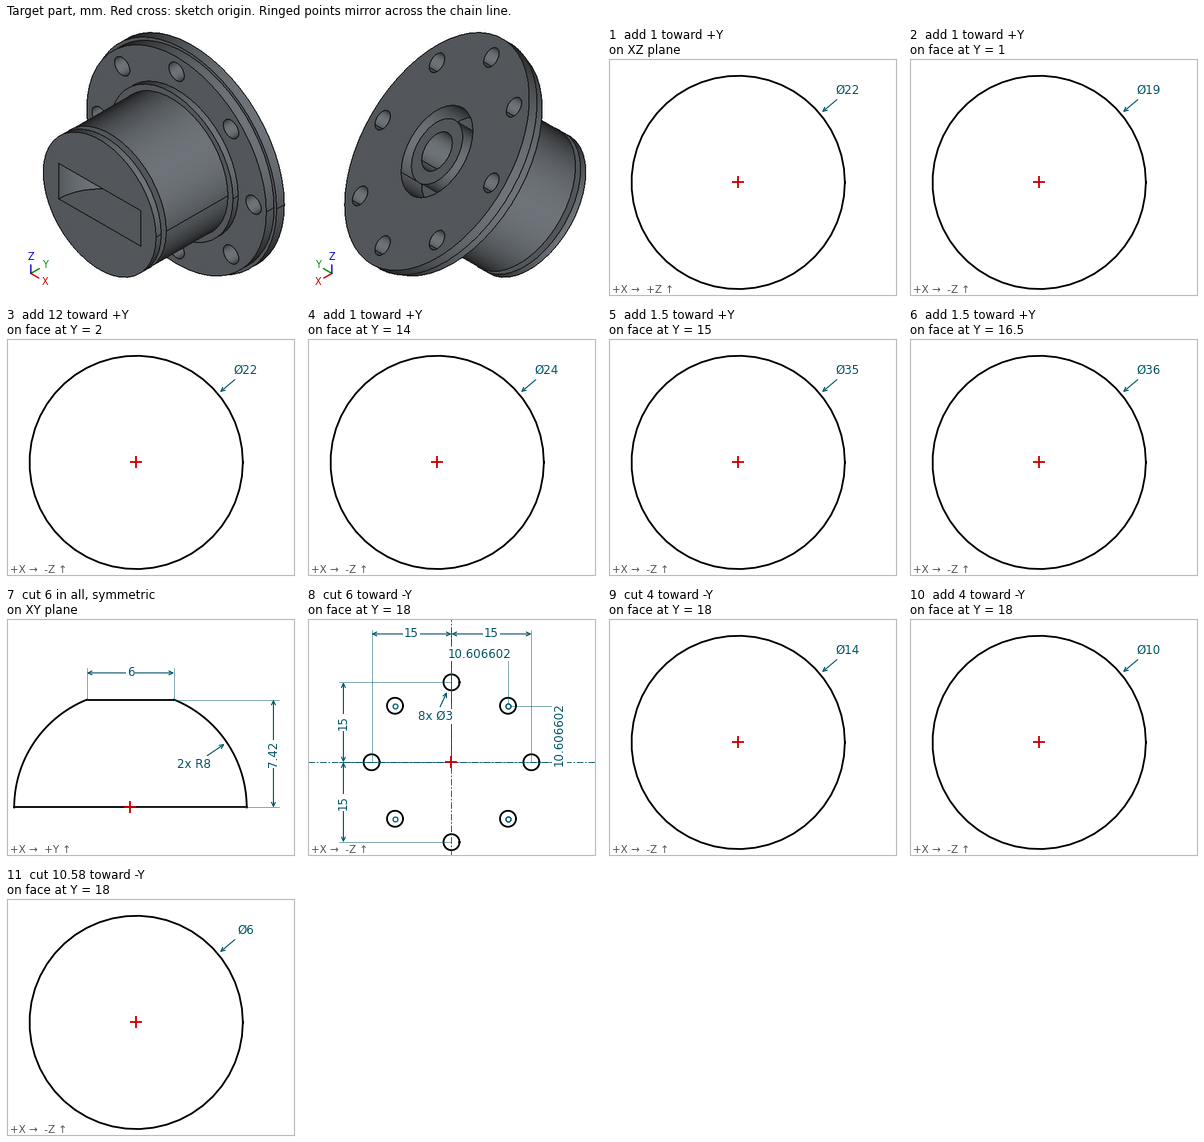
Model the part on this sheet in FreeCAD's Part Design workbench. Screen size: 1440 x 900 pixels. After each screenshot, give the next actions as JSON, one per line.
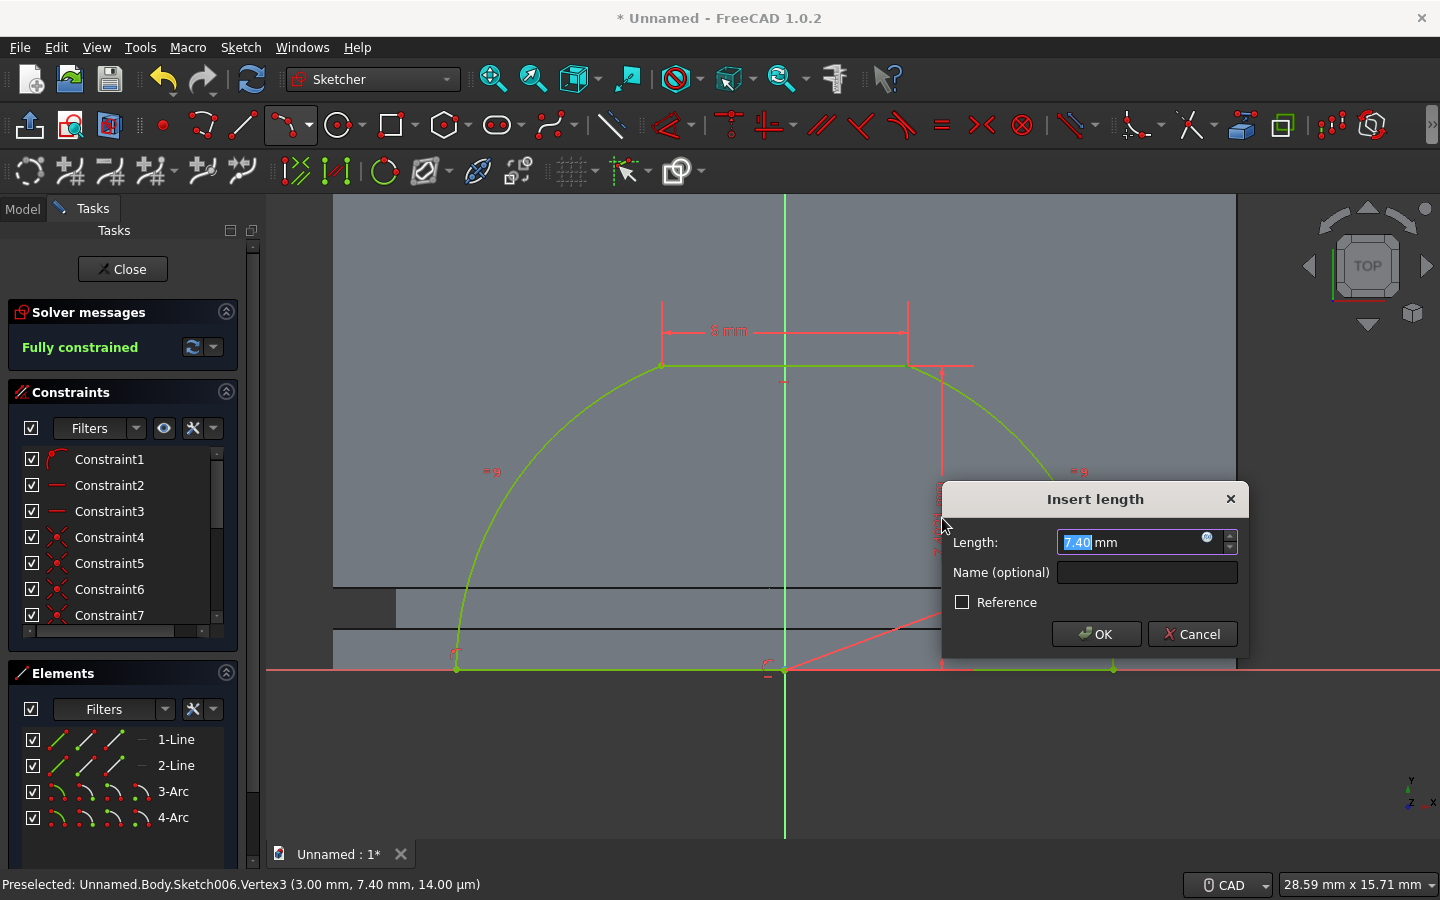
{"action": "type", "text": "7.42"}
{"action": "key", "text": "Return"}
{"action": "key", "text": "Escape"}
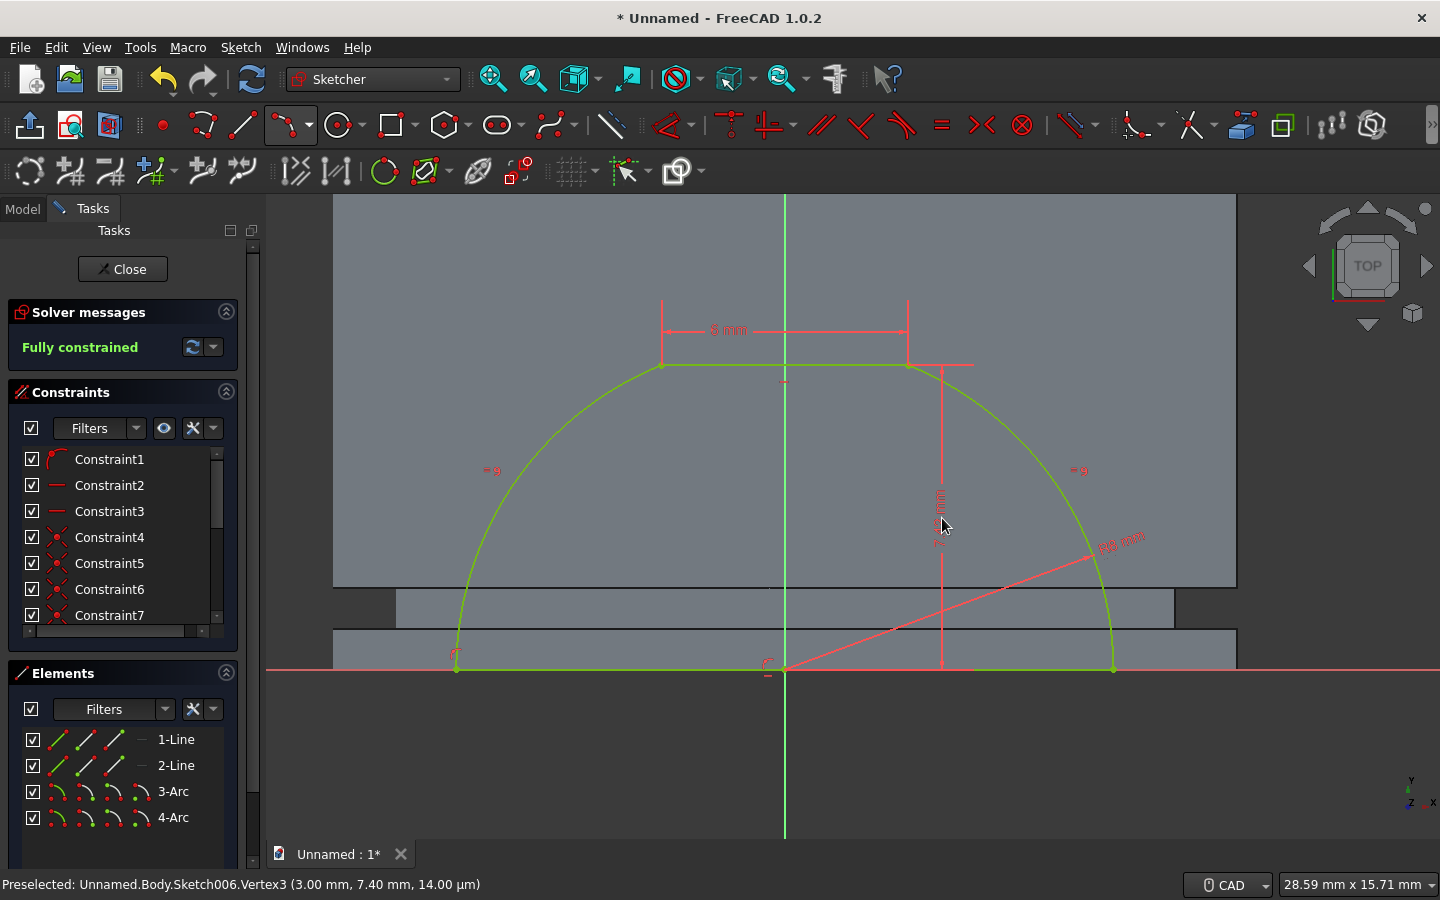
{"action": "left_click", "coordinate": [123, 269]}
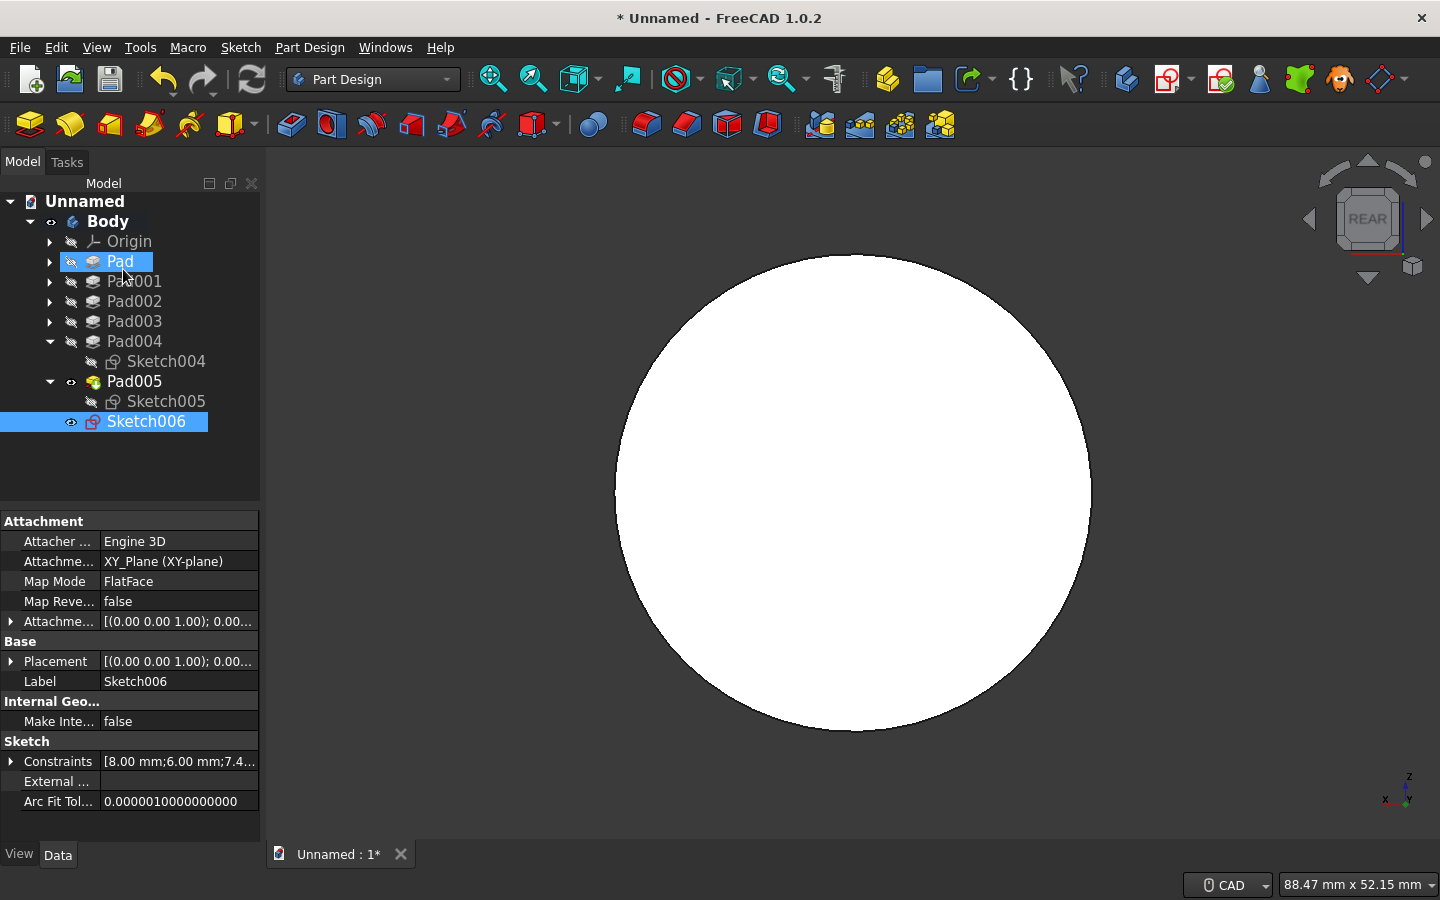
{"action": "left_click", "coordinate": [292, 124]}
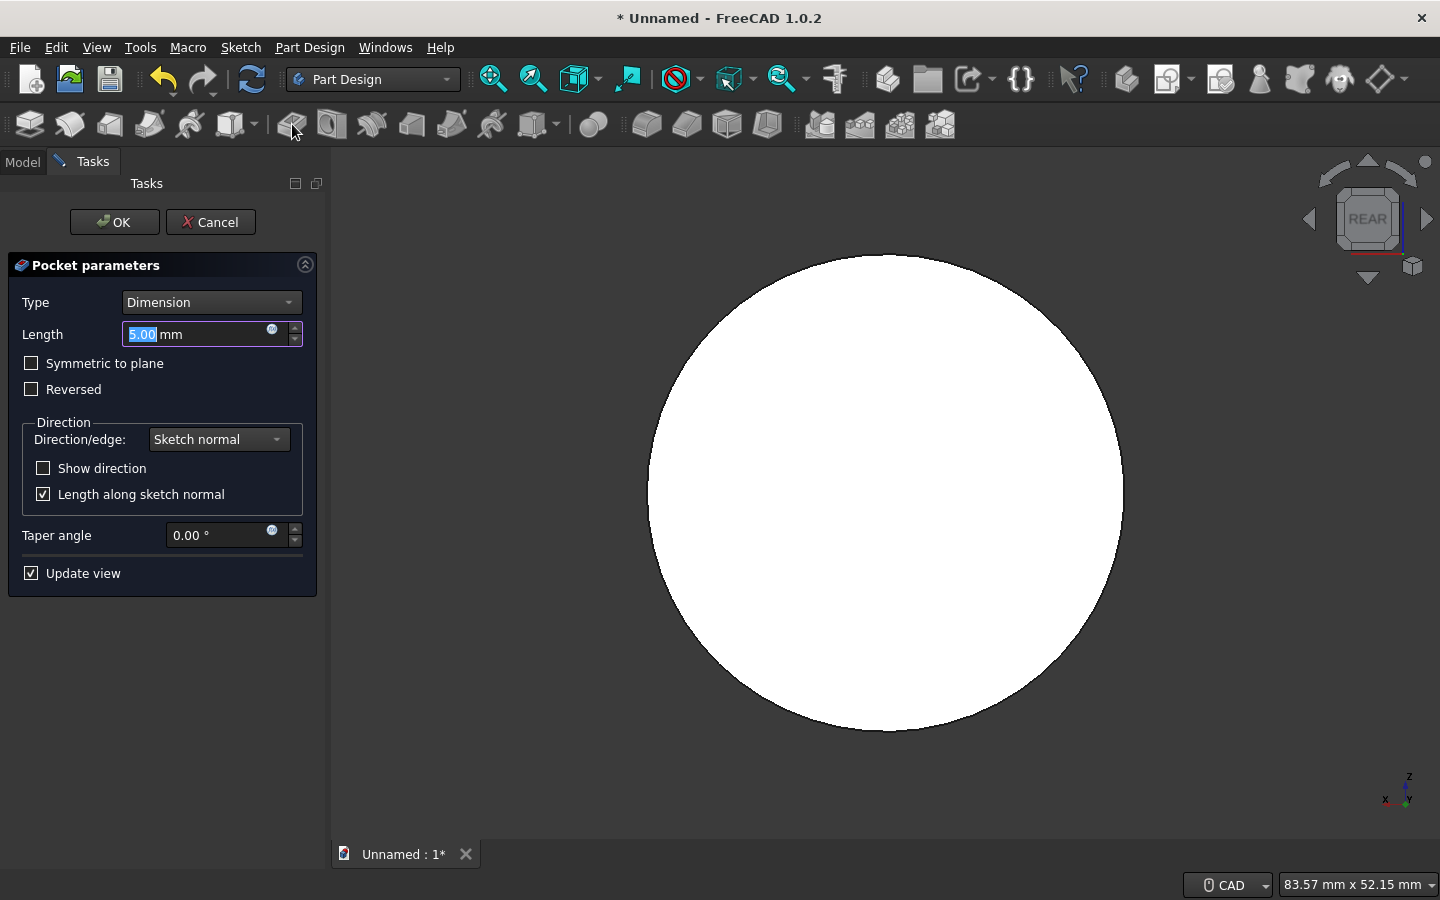
{"action": "type", "text": "6"}
{"action": "key", "text": "Tab"}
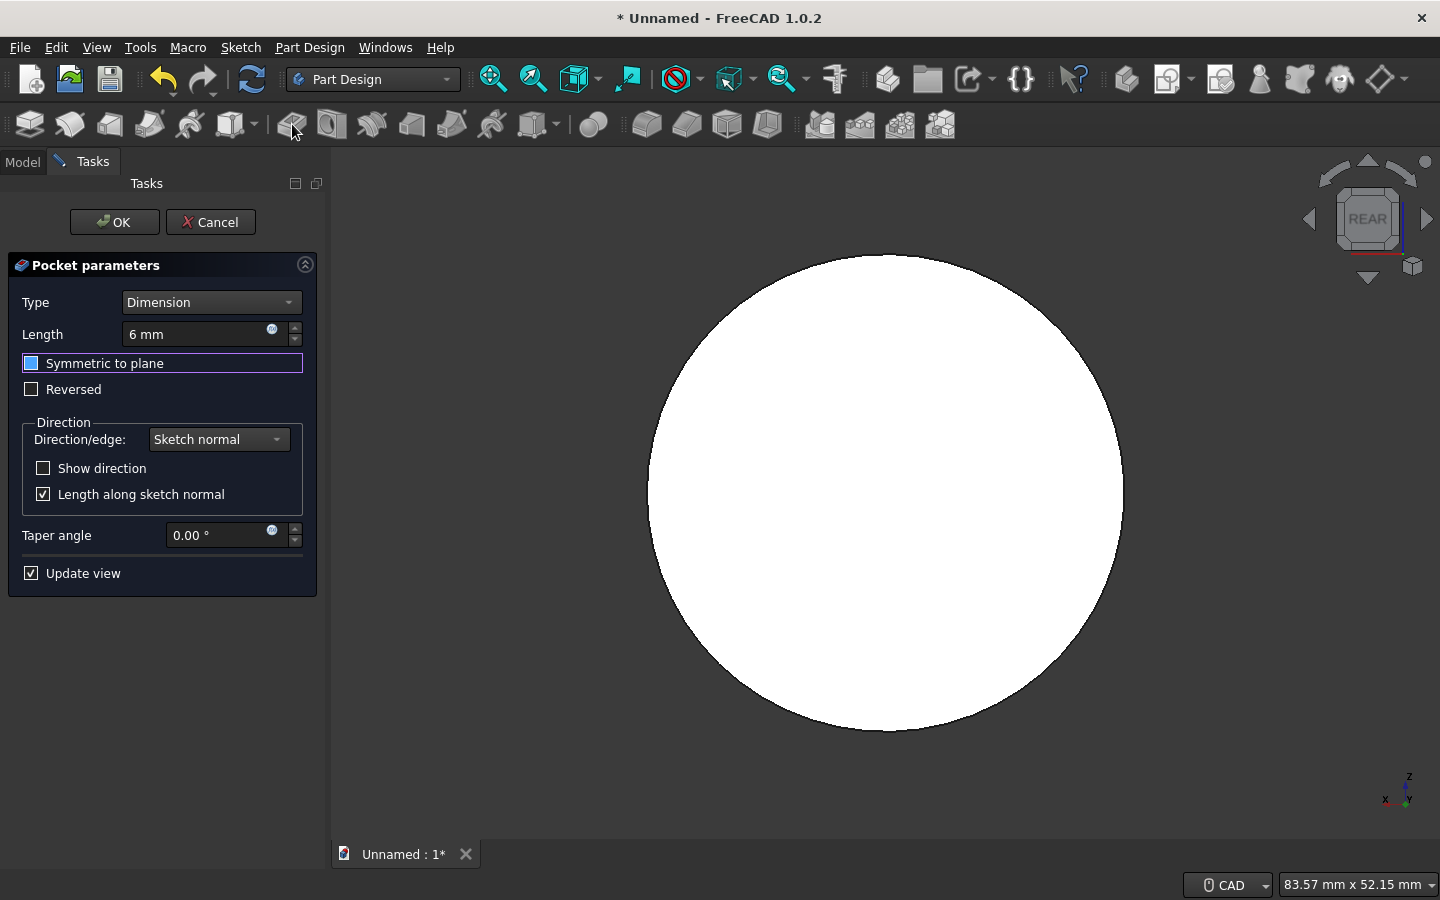
{"action": "left_click", "coordinate": [30, 363]}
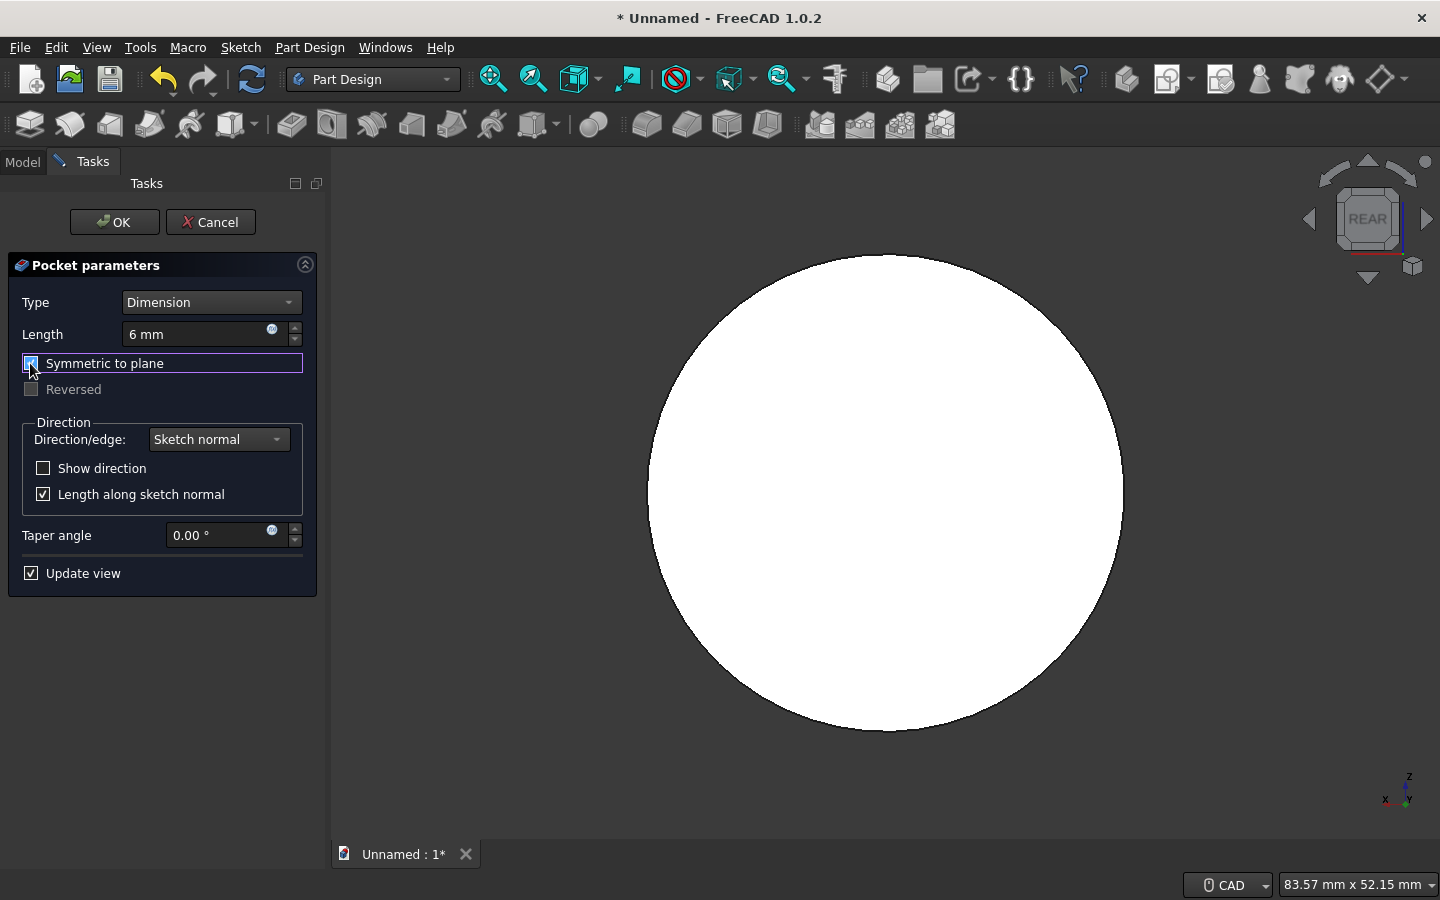
{"action": "left_click", "coordinate": [115, 222]}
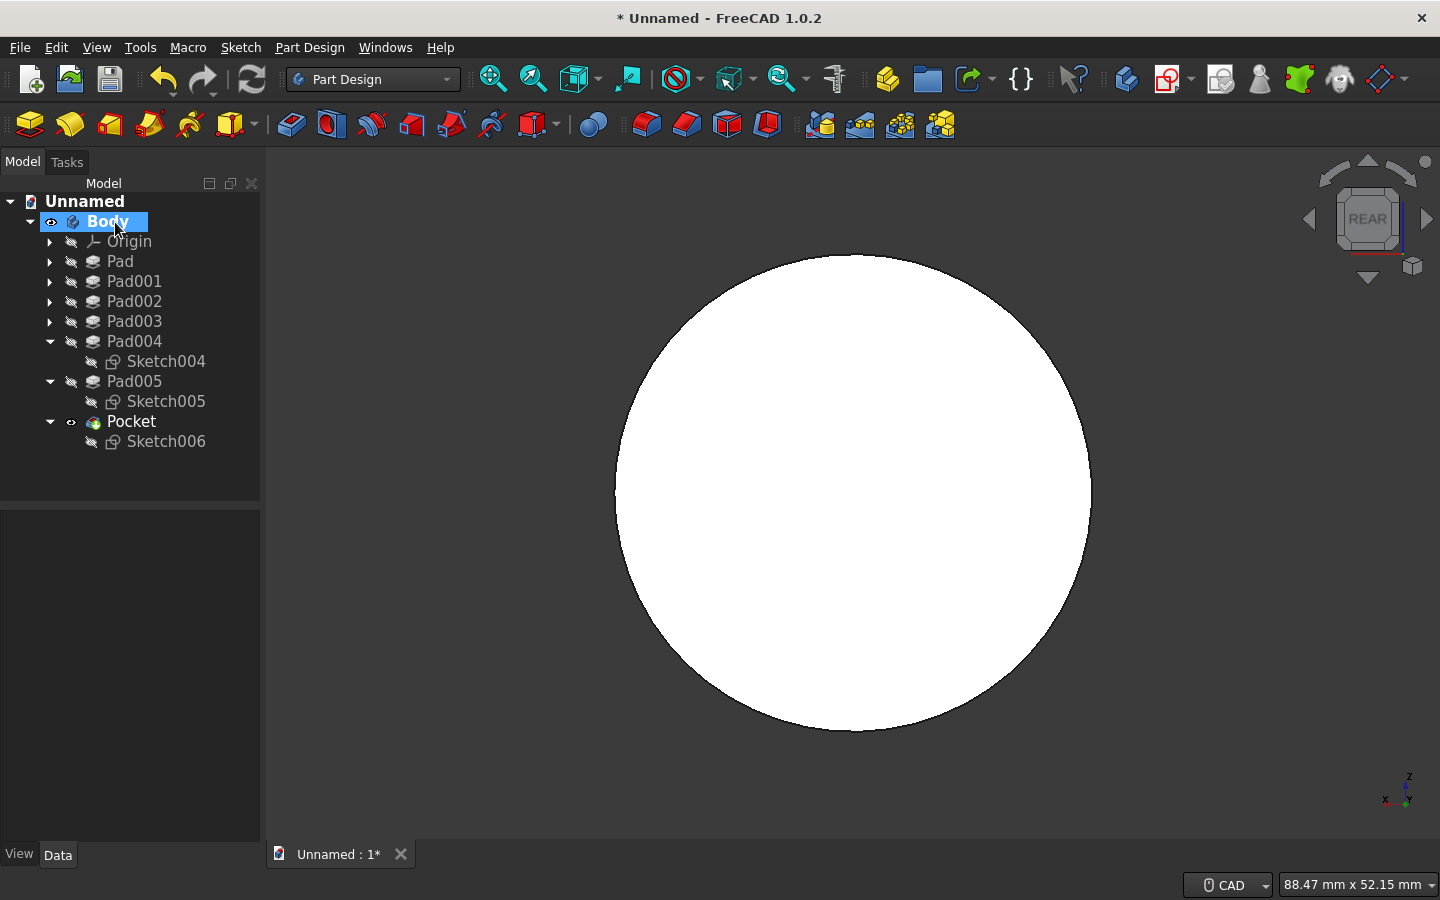
{"action": "left_click", "coordinate": [853, 492]}